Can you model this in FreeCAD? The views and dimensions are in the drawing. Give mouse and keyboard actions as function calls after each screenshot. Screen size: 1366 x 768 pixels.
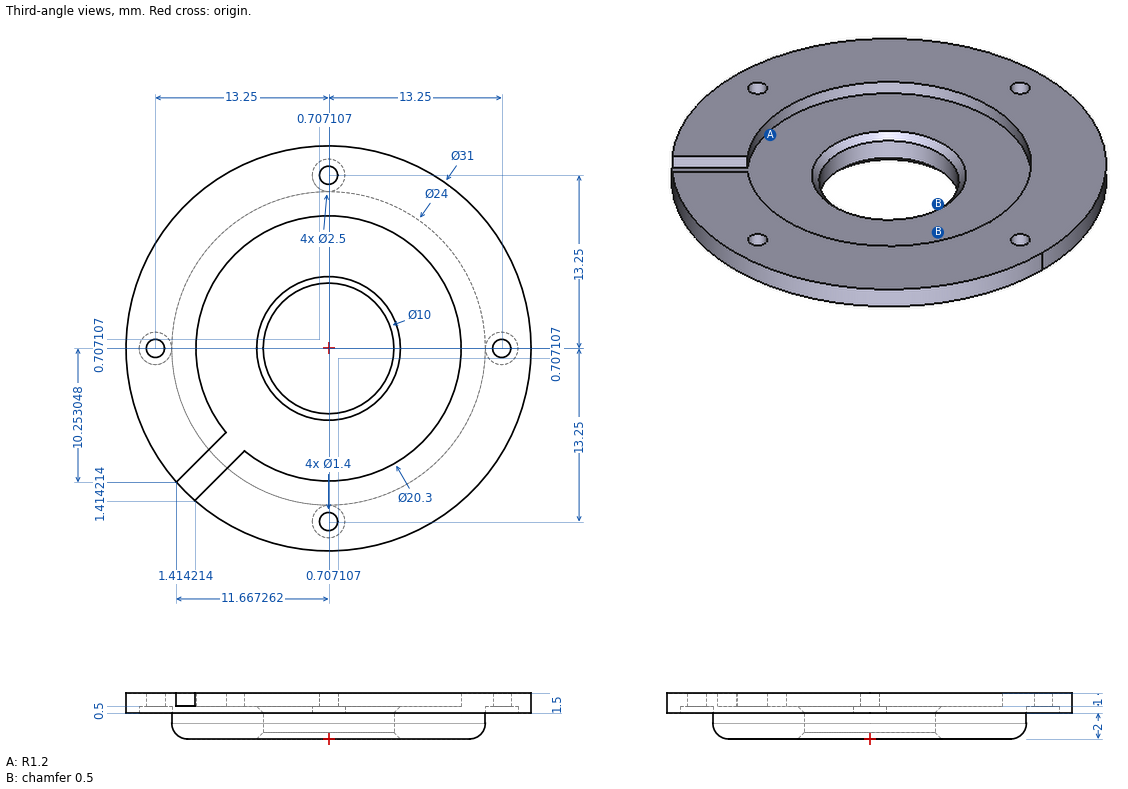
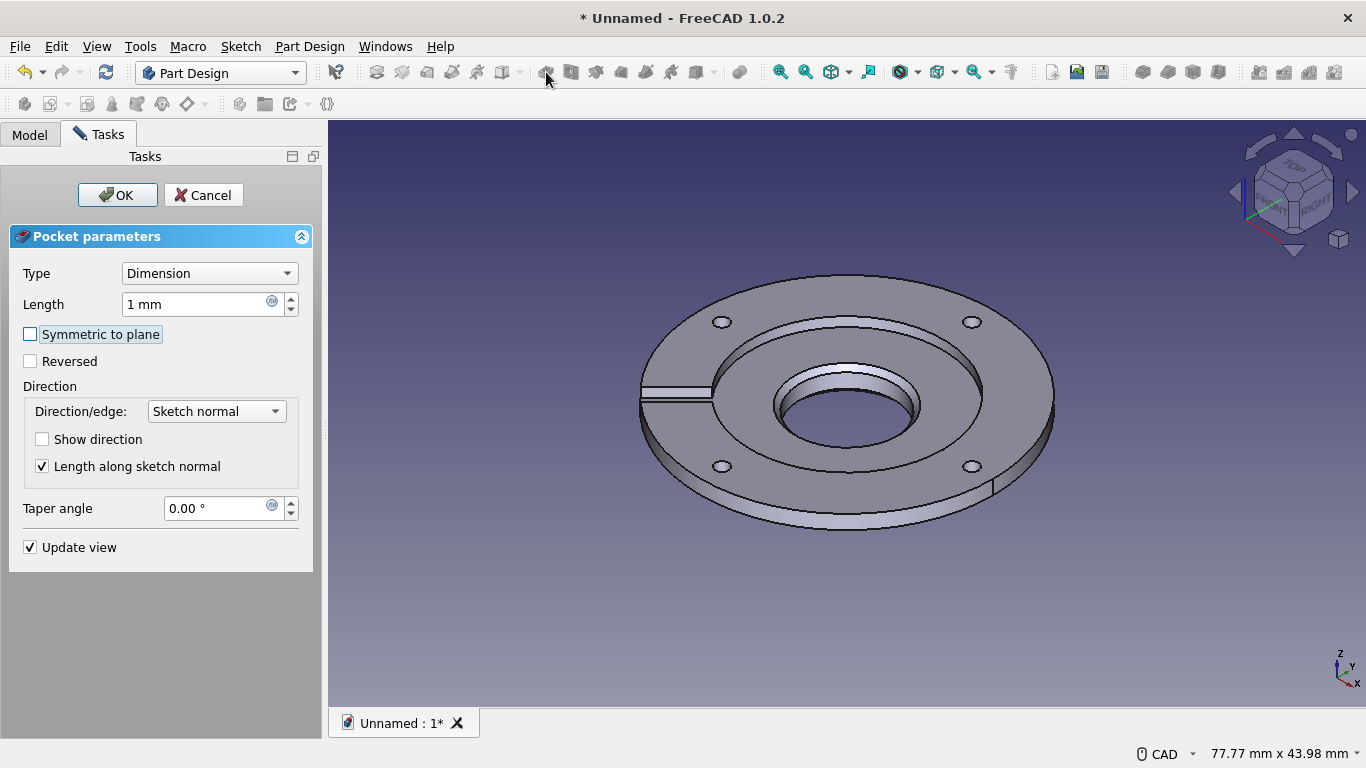
click(118, 195)